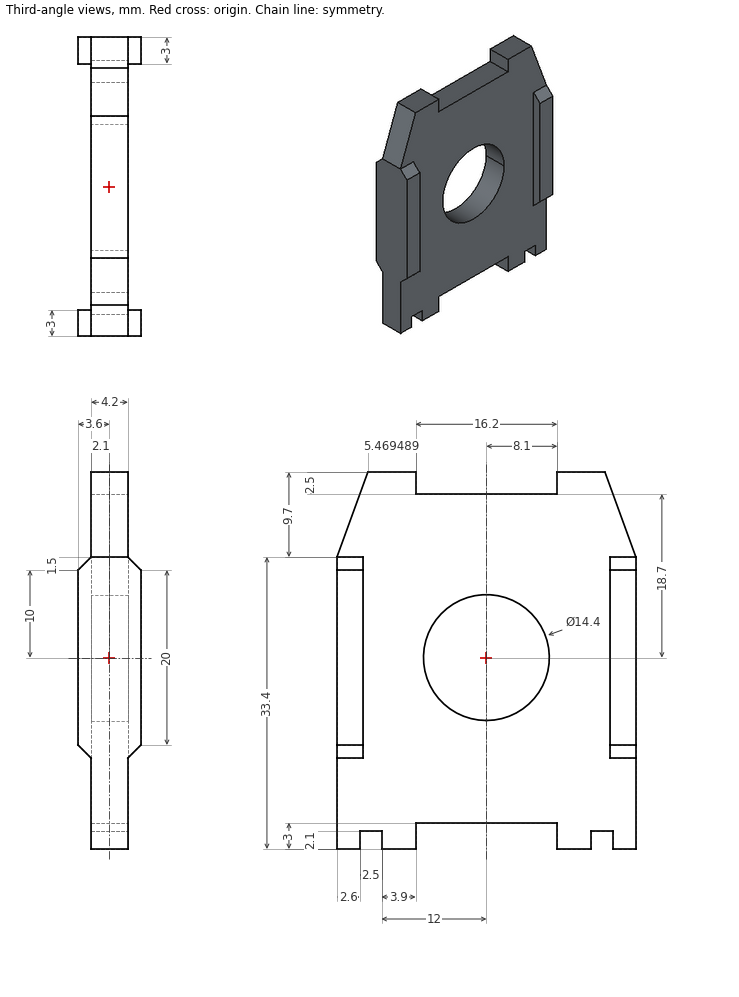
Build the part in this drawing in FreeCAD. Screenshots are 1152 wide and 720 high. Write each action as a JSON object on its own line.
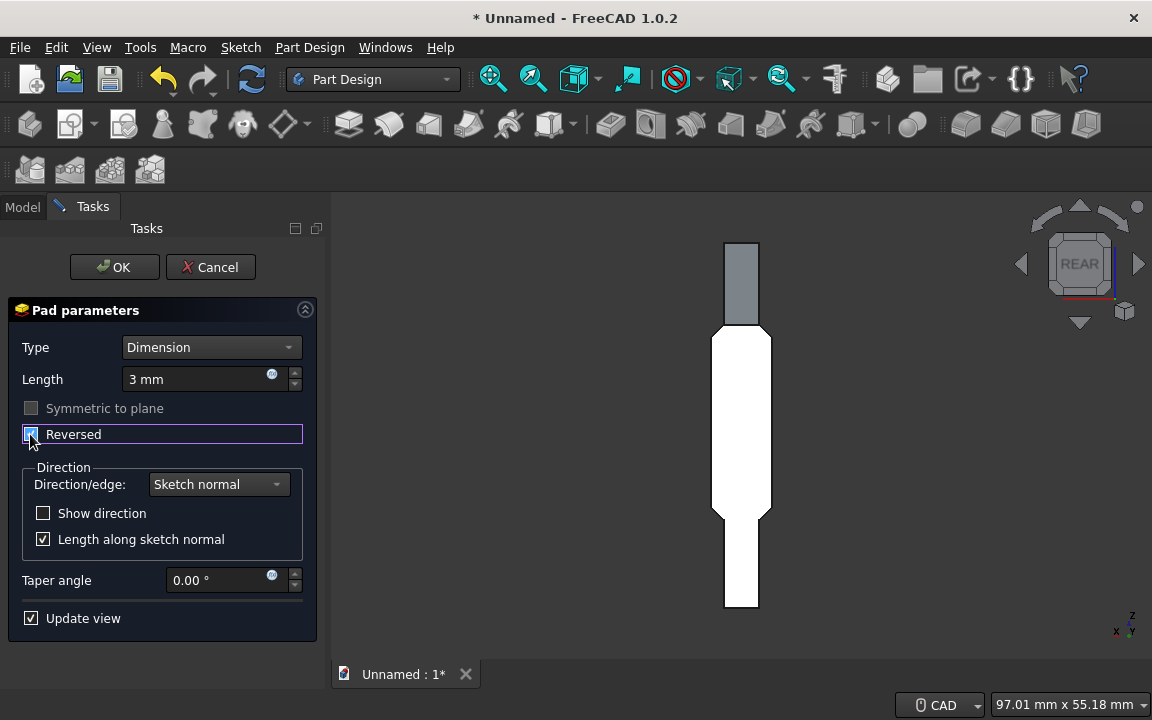
{"action": "left_click", "coordinate": [115, 267]}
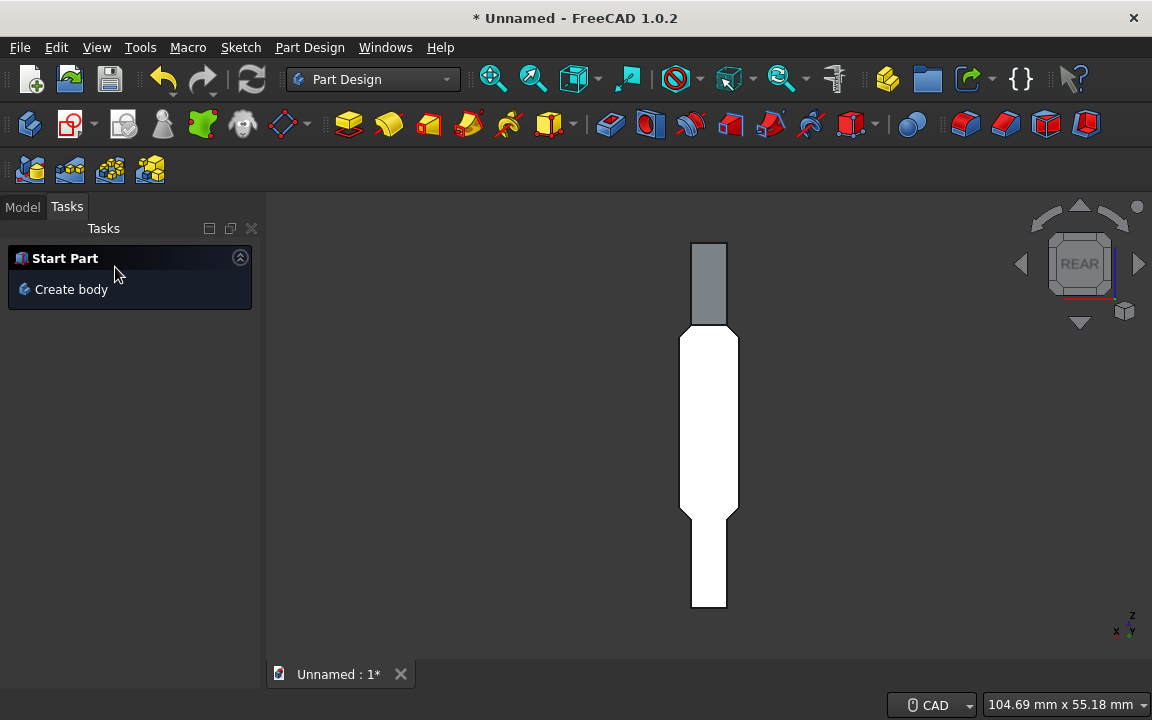
{"action": "key", "text": "0"}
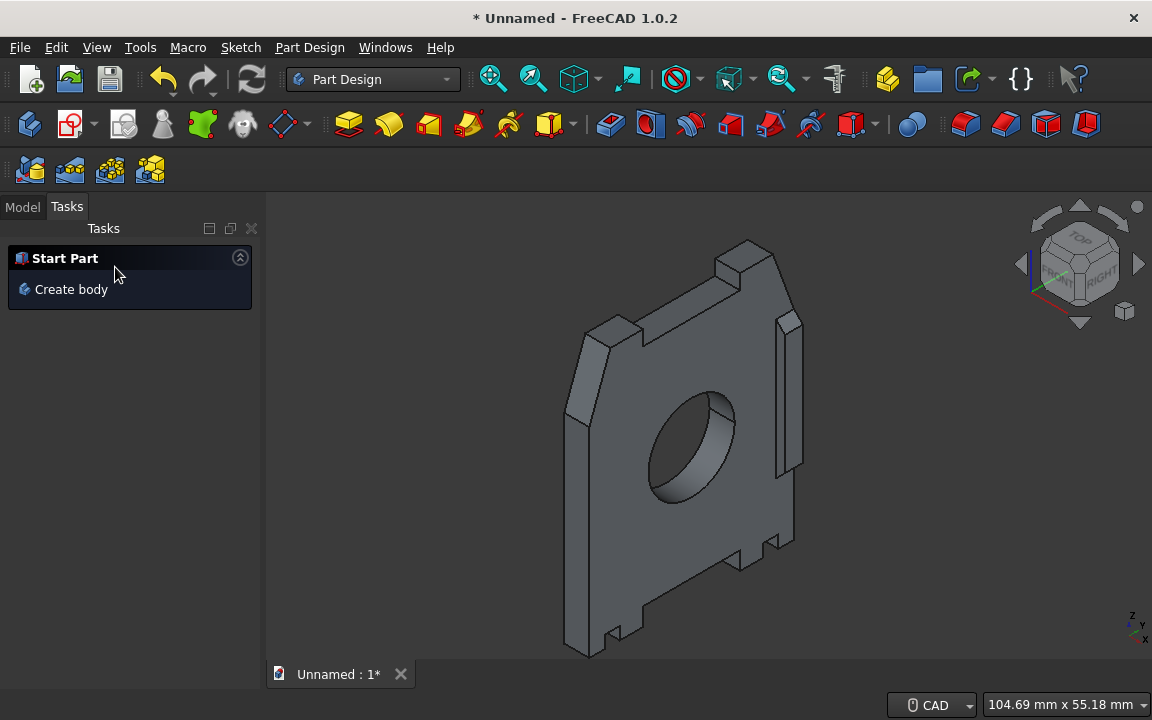
{"action": "left_click", "coordinate": [494, 80]}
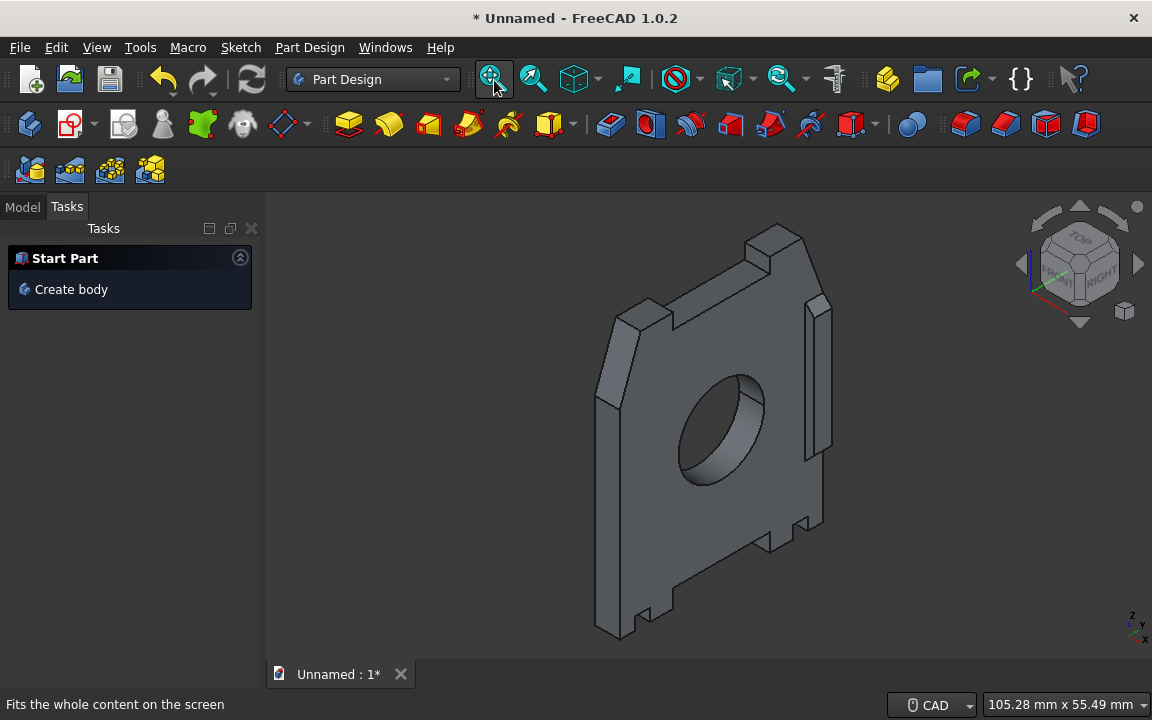
{"action": "left_click", "coordinate": [607, 615]}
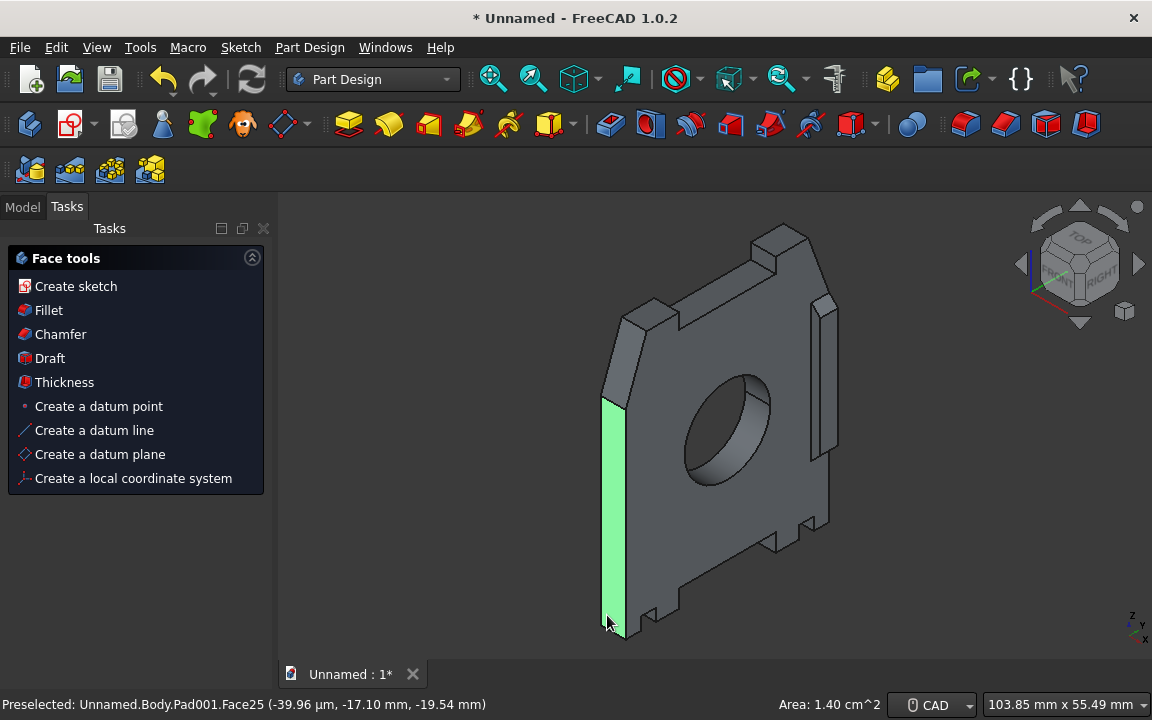
{"action": "left_click", "coordinate": [70, 124]}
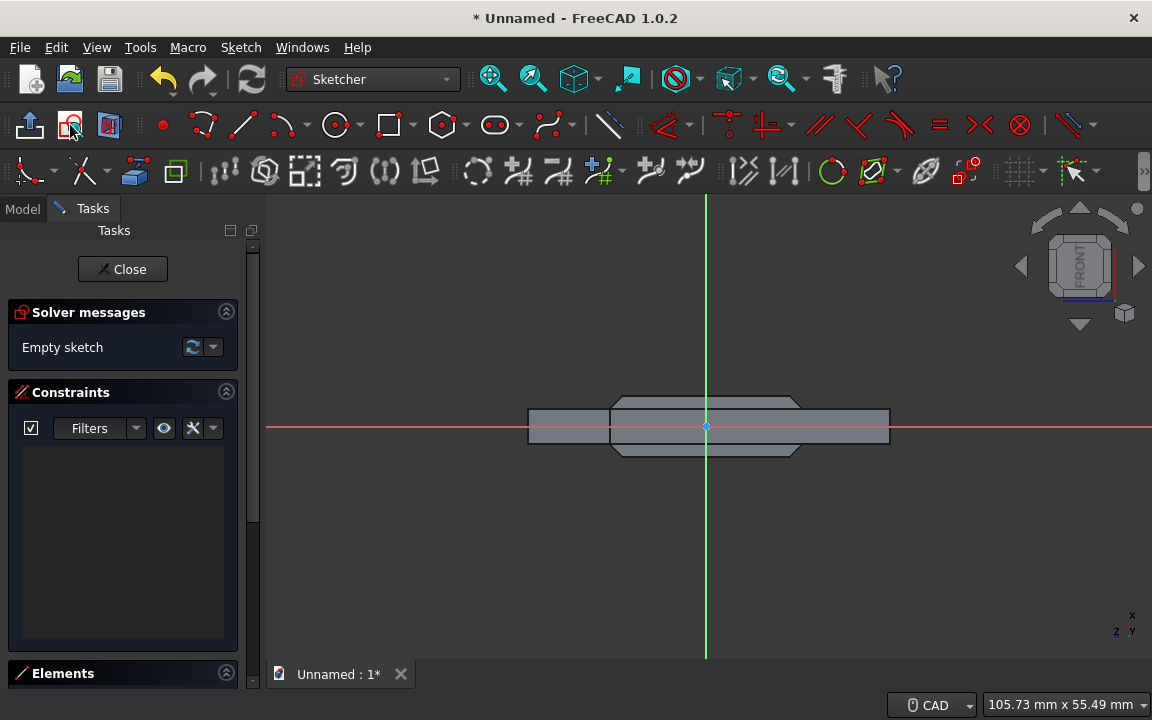
{"action": "scroll", "coordinate": [744, 427], "scroll_direction": "up", "scroll_amount": 5}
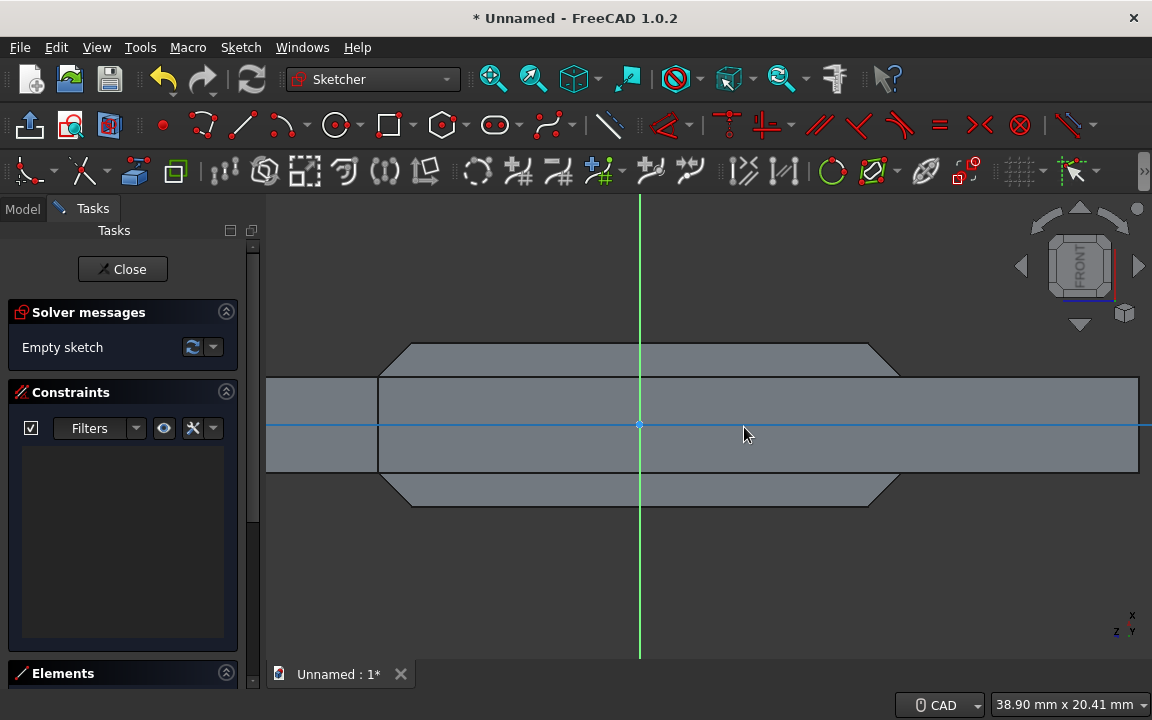
{"action": "left_click", "coordinate": [204, 126]}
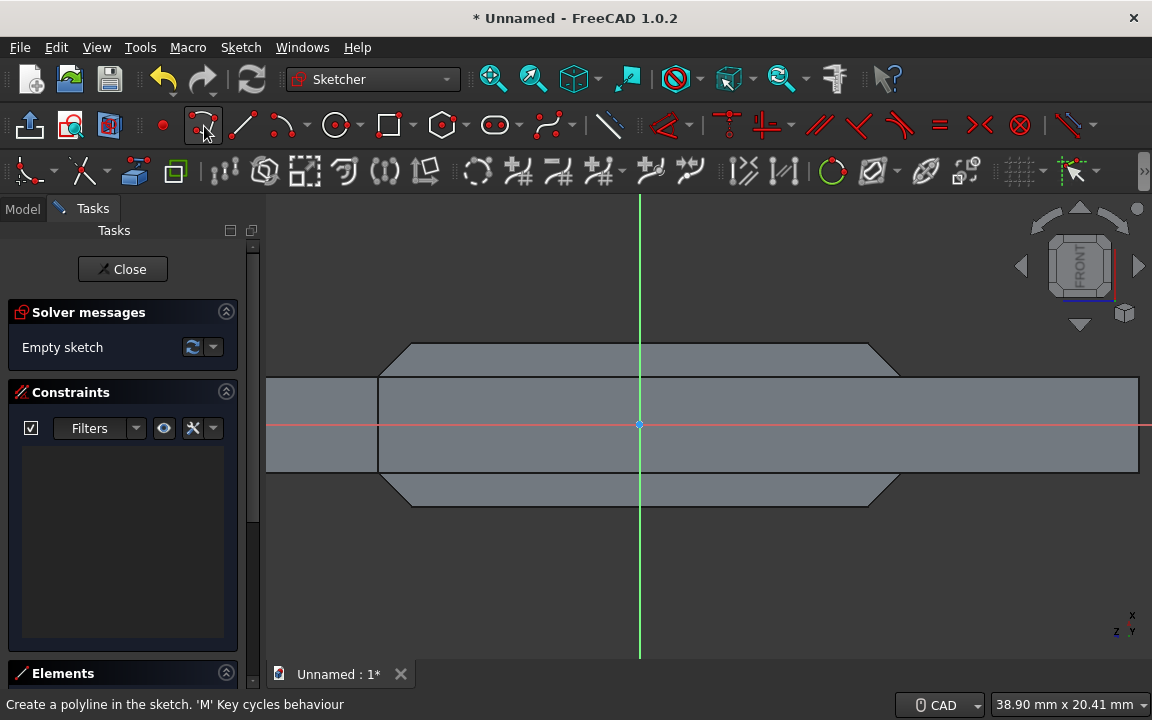
{"action": "left_click", "coordinate": [412, 507]}
{"action": "left_click", "coordinate": [378, 473]}
{"action": "left_click", "coordinate": [378, 377]}
{"action": "left_click", "coordinate": [412, 343]}
{"action": "left_click", "coordinate": [868, 343]}
{"action": "left_click", "coordinate": [902, 377]}
{"action": "left_click", "coordinate": [902, 473]}
{"action": "left_click", "coordinate": [868, 507]}
{"action": "left_click", "coordinate": [412, 508]}
{"action": "key", "text": "Escape"}
{"action": "key", "text": "Escape"}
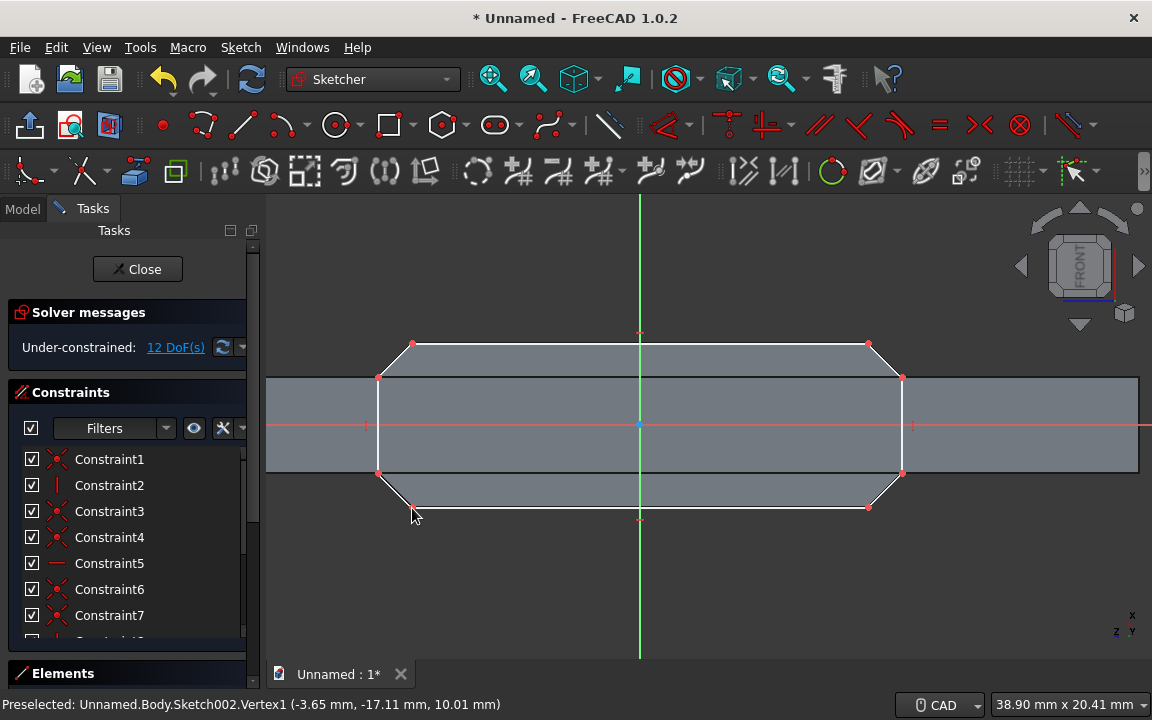
{"action": "left_click", "coordinate": [412, 508]}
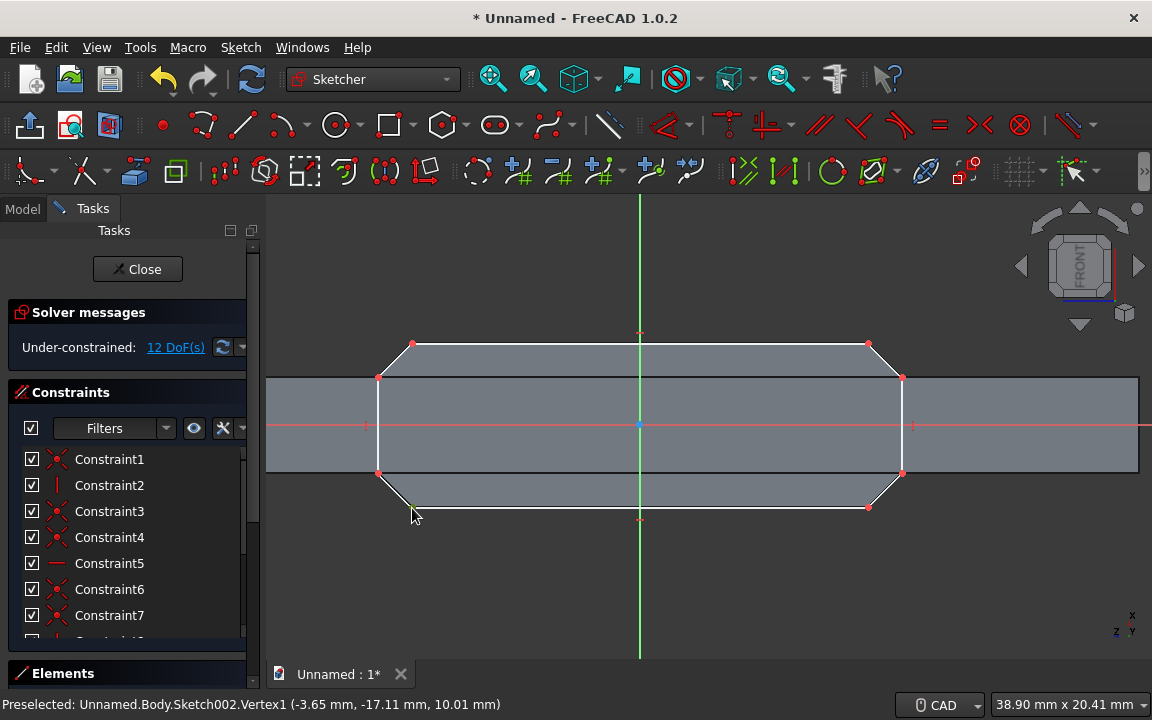
{"action": "left_click", "coordinate": [412, 344]}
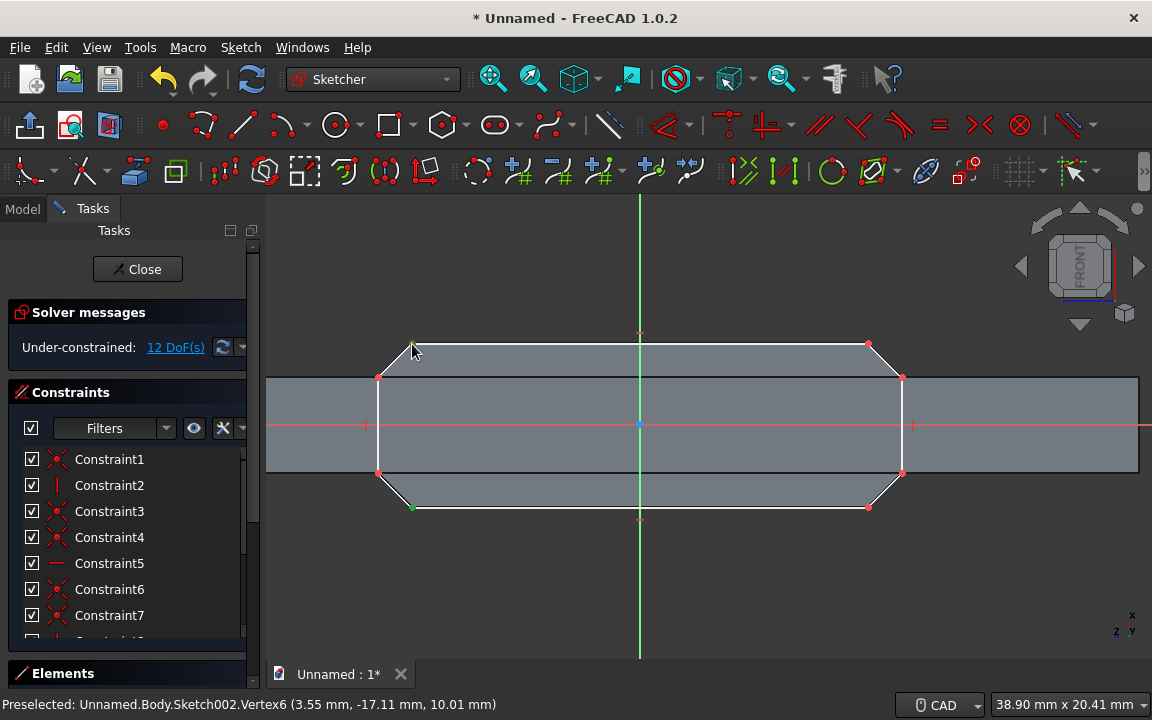
{"action": "left_click", "coordinate": [344, 425]}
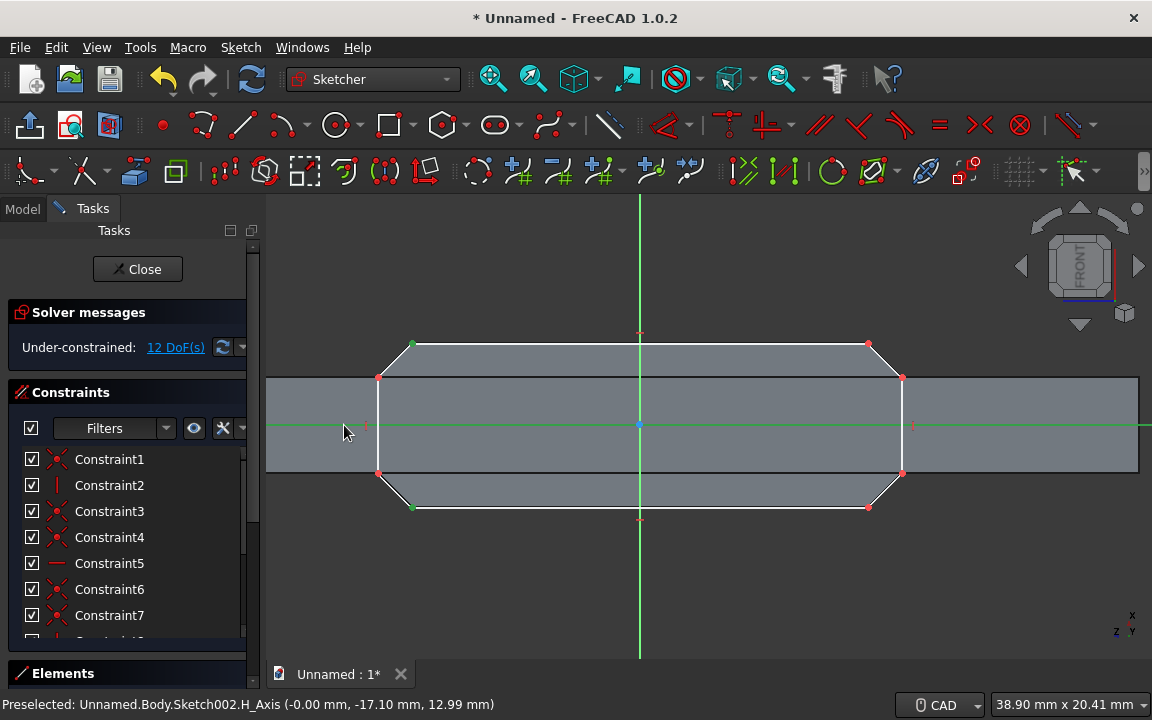
{"action": "left_click", "coordinate": [980, 126]}